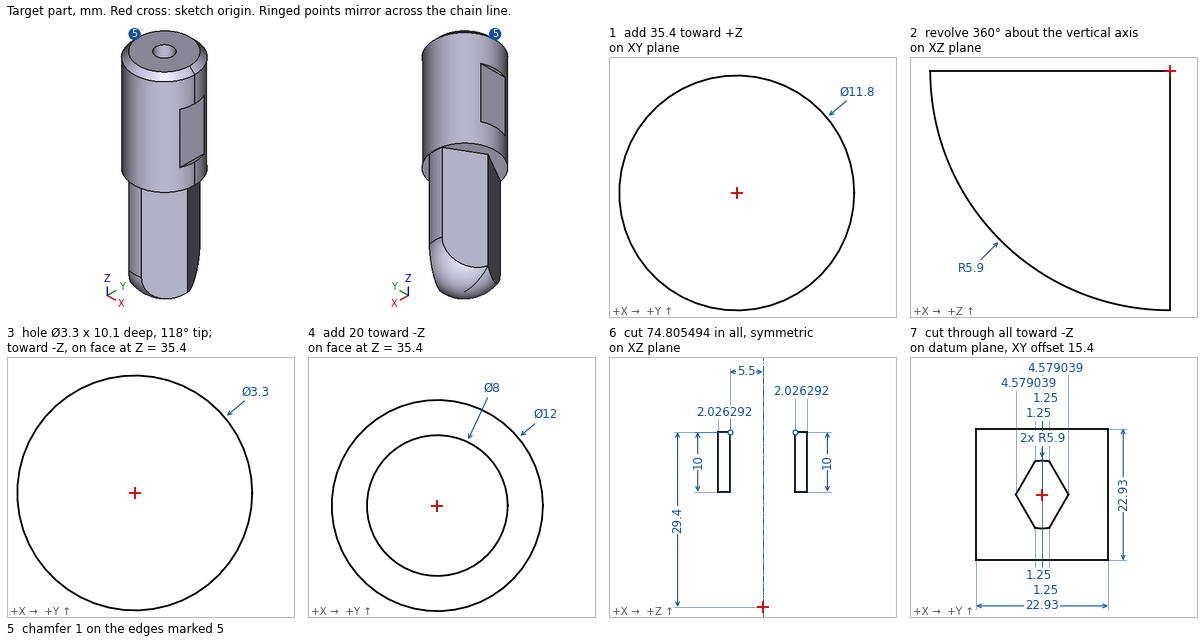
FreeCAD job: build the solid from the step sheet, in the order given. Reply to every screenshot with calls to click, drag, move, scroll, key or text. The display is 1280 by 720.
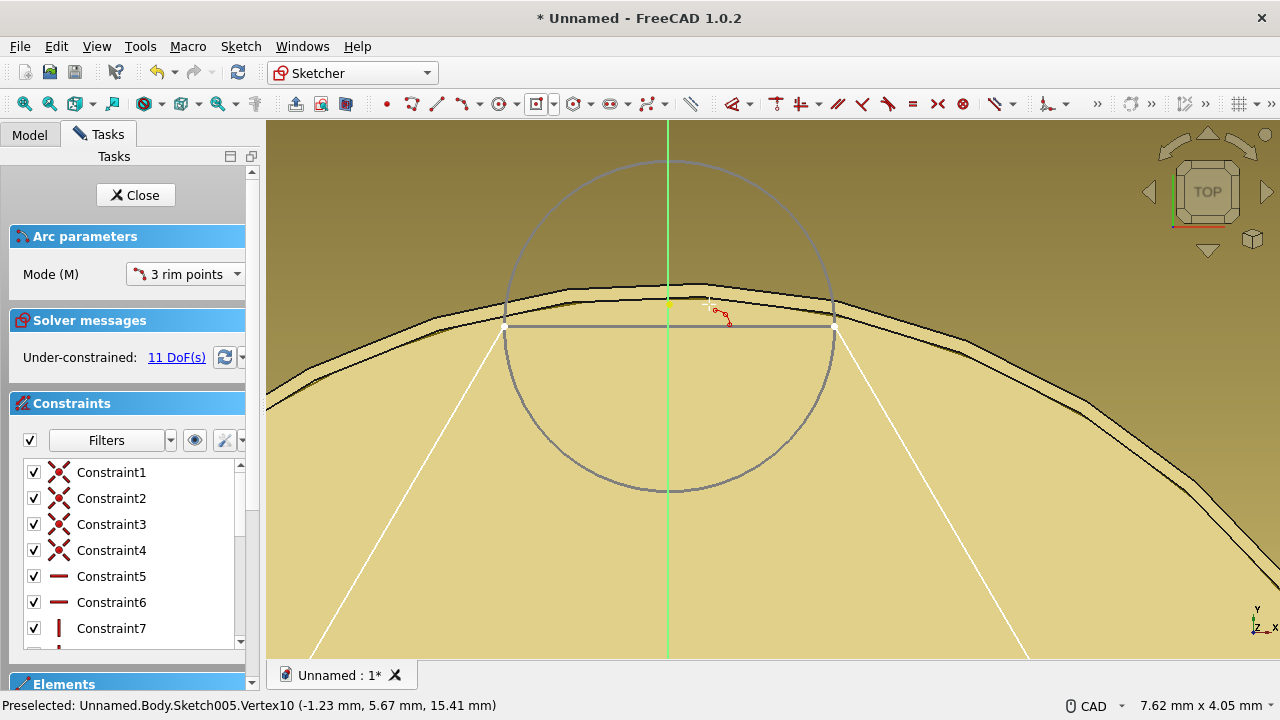
click(702, 297)
key(Escape)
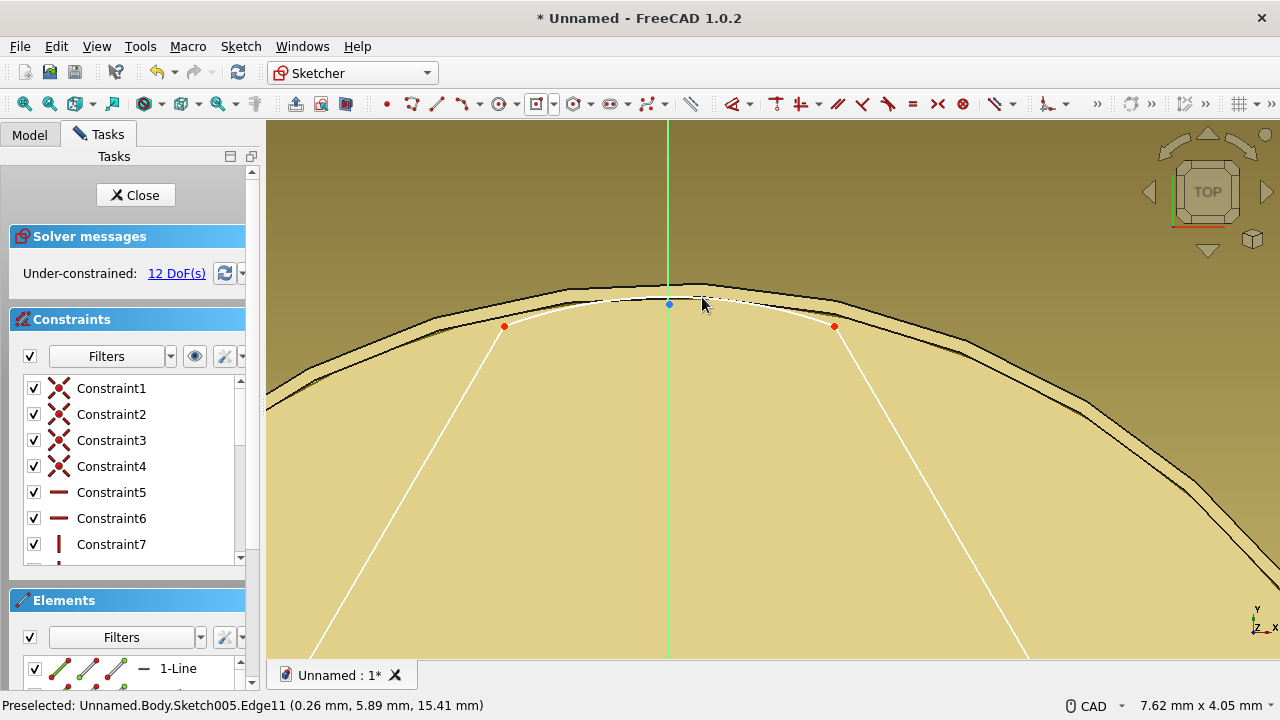
scroll(709, 303, down, 11)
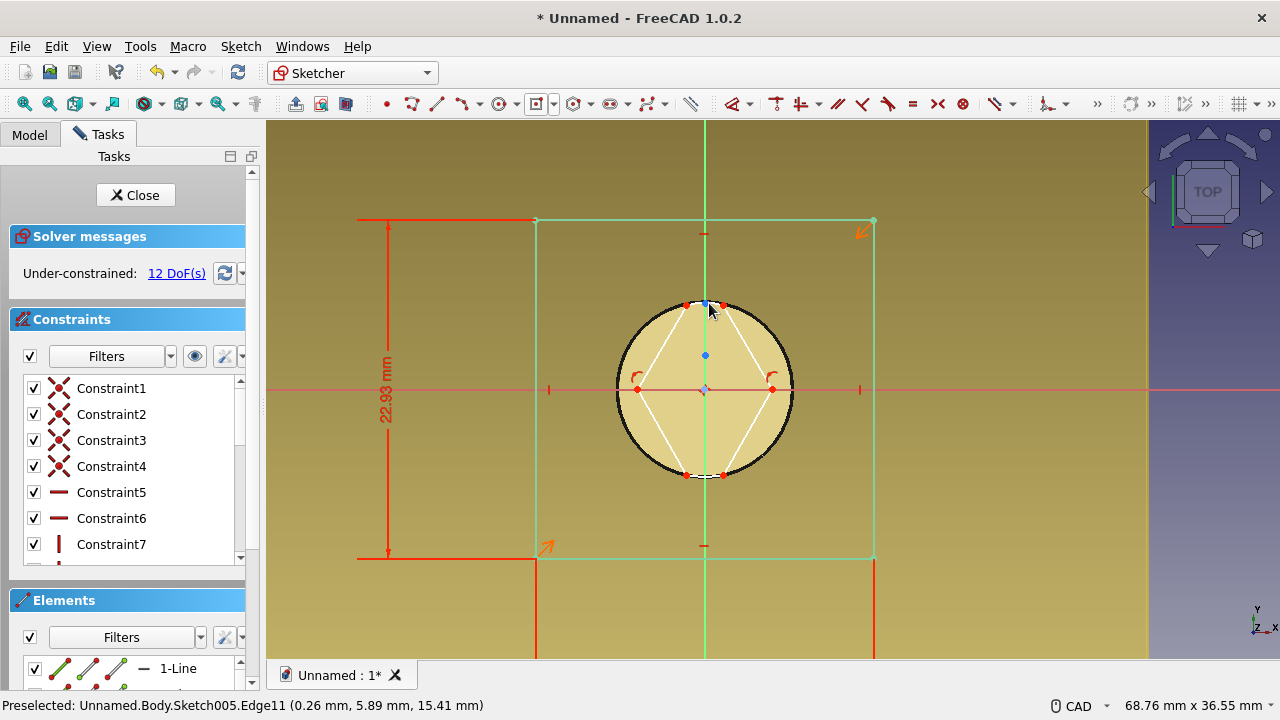
scroll(698, 476, up, 4)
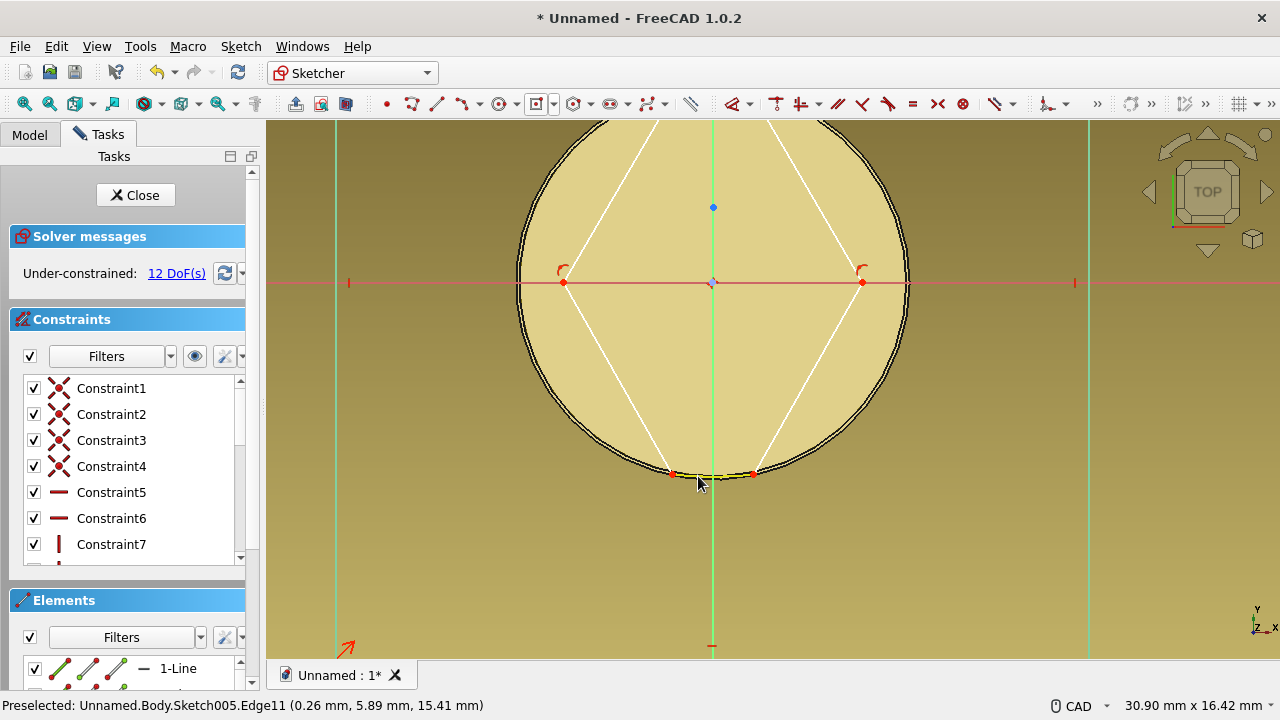
click(697, 476)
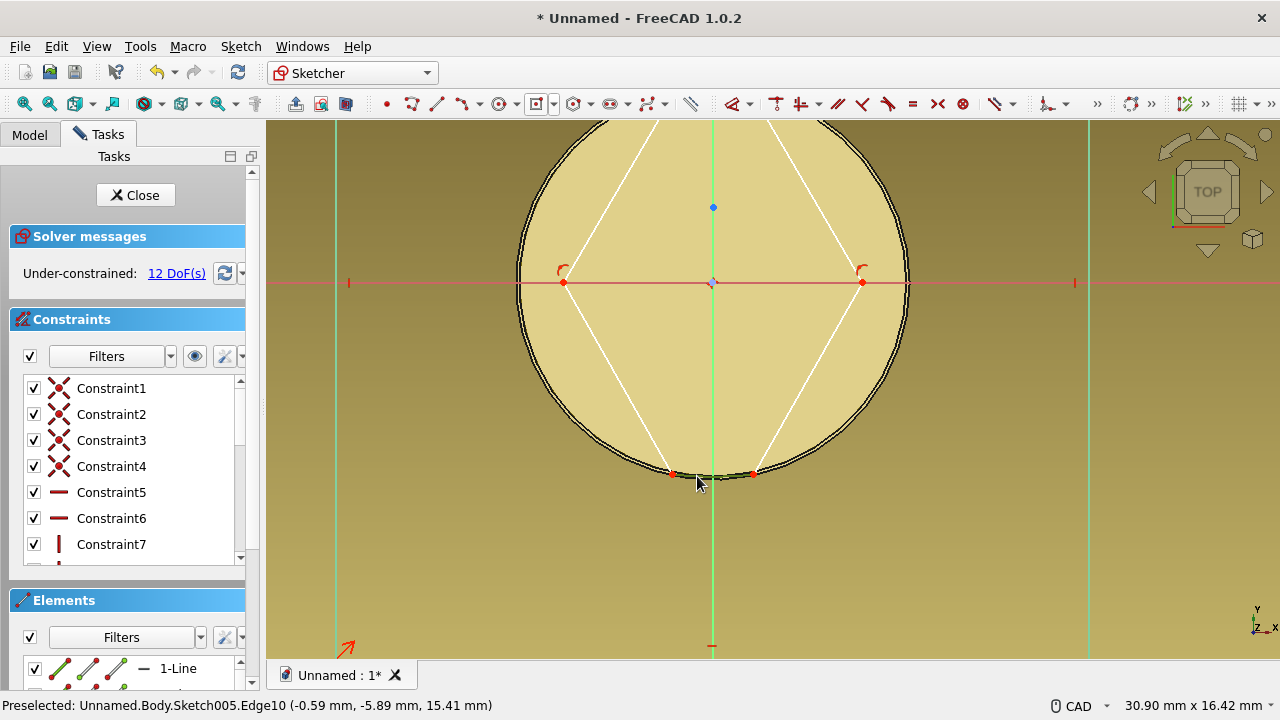
scroll(698, 477, down, 4)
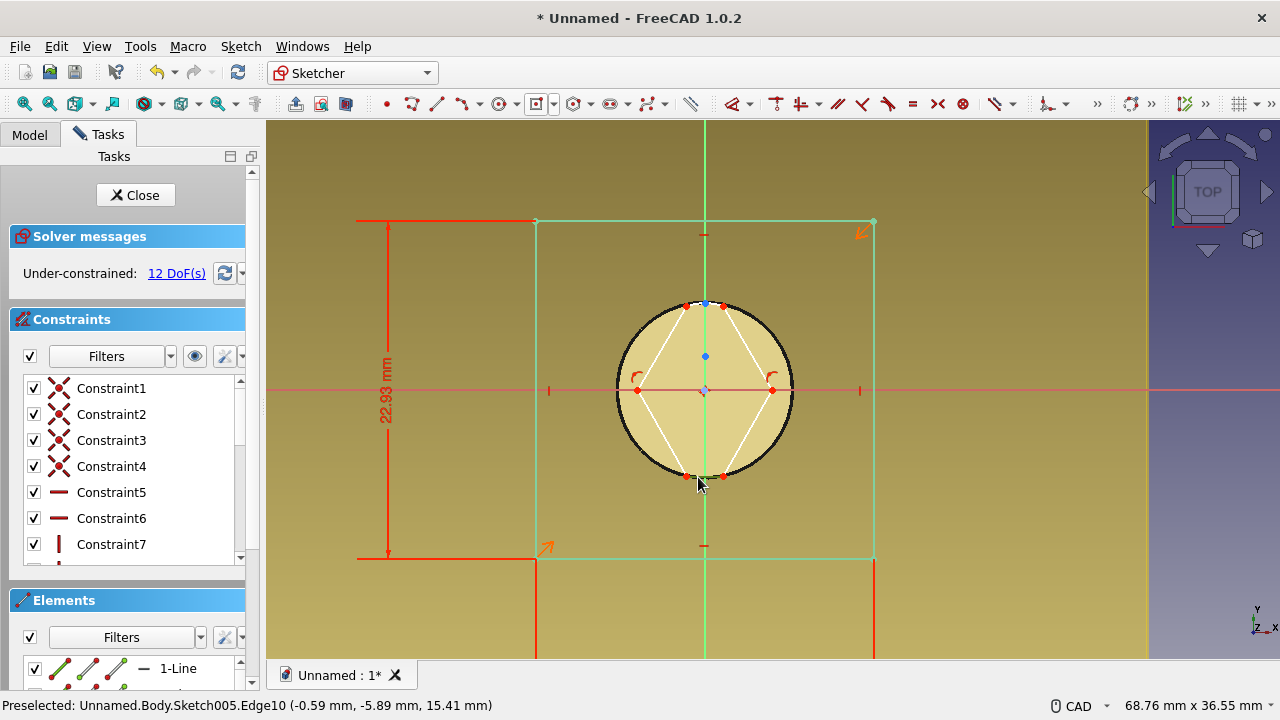
scroll(712, 304, up, 3)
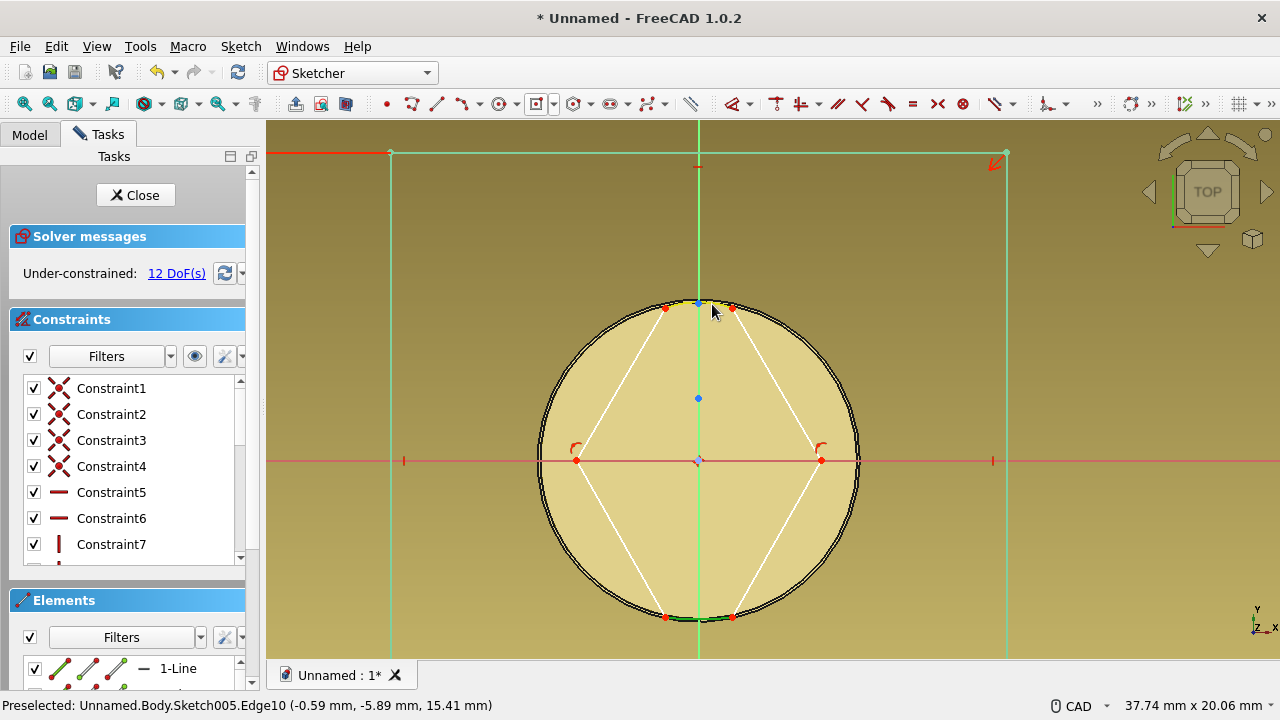
click(713, 303)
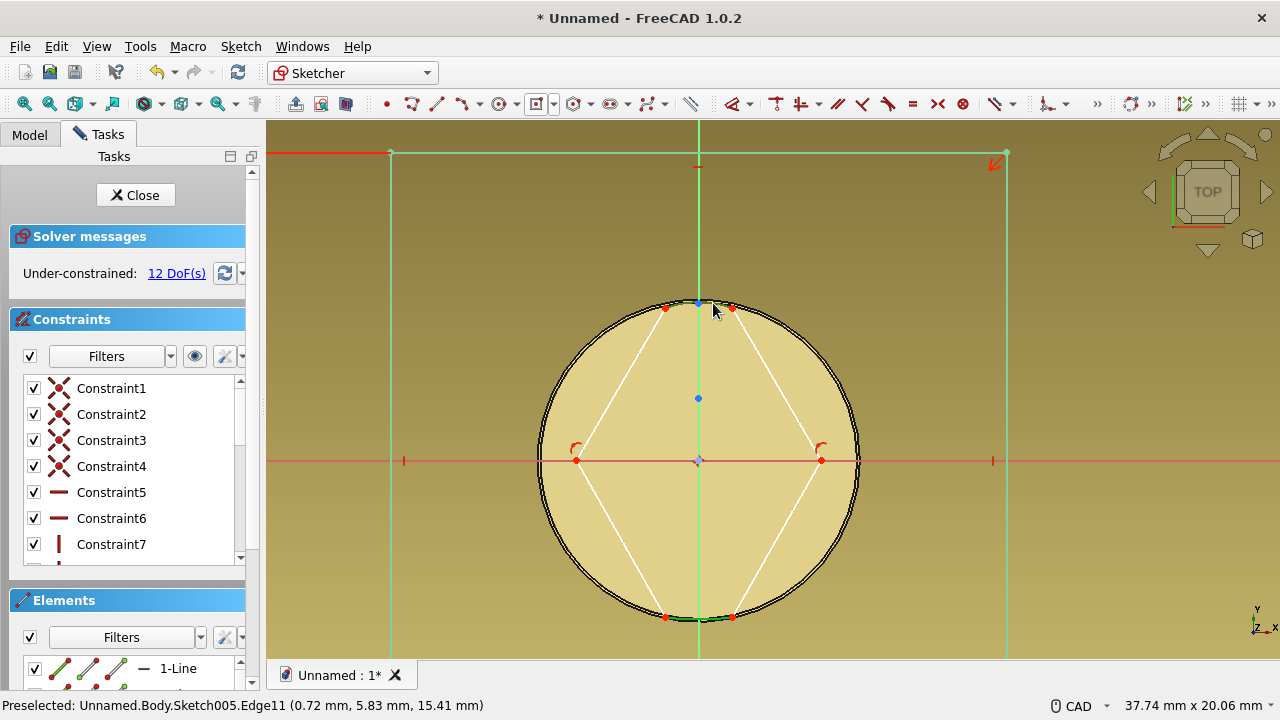
key(c)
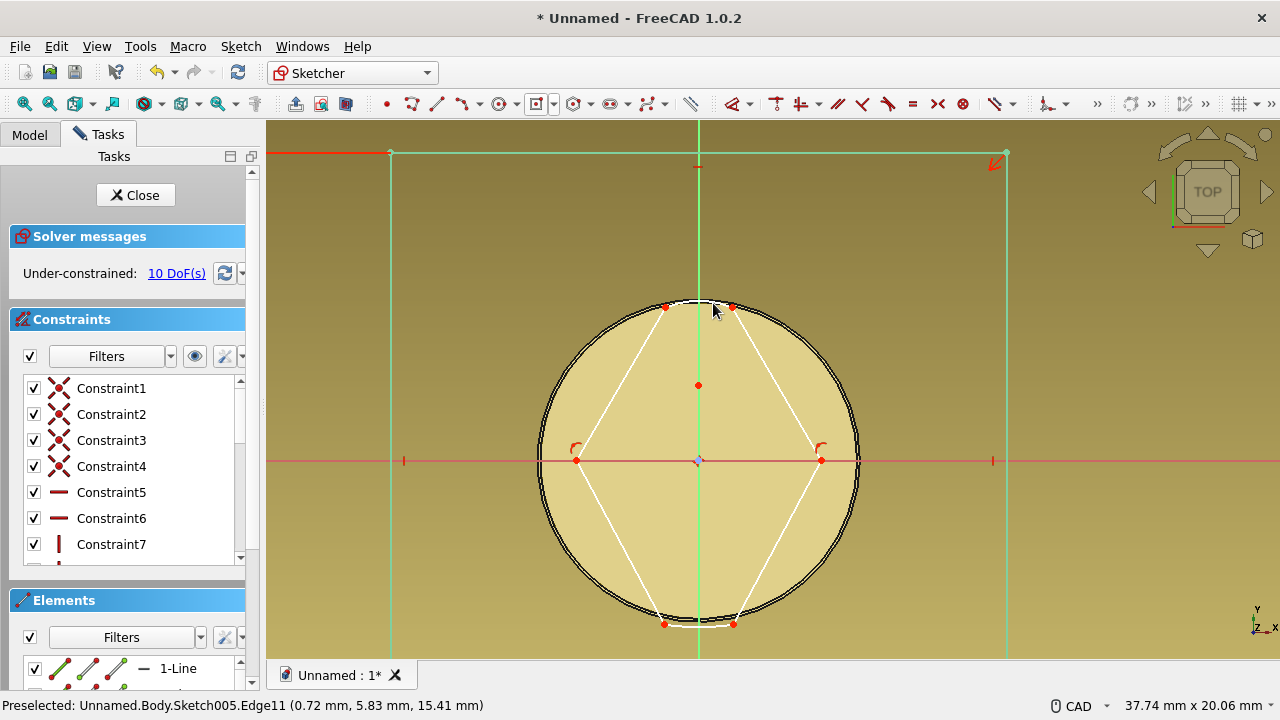
drag(689, 375, 709, 471)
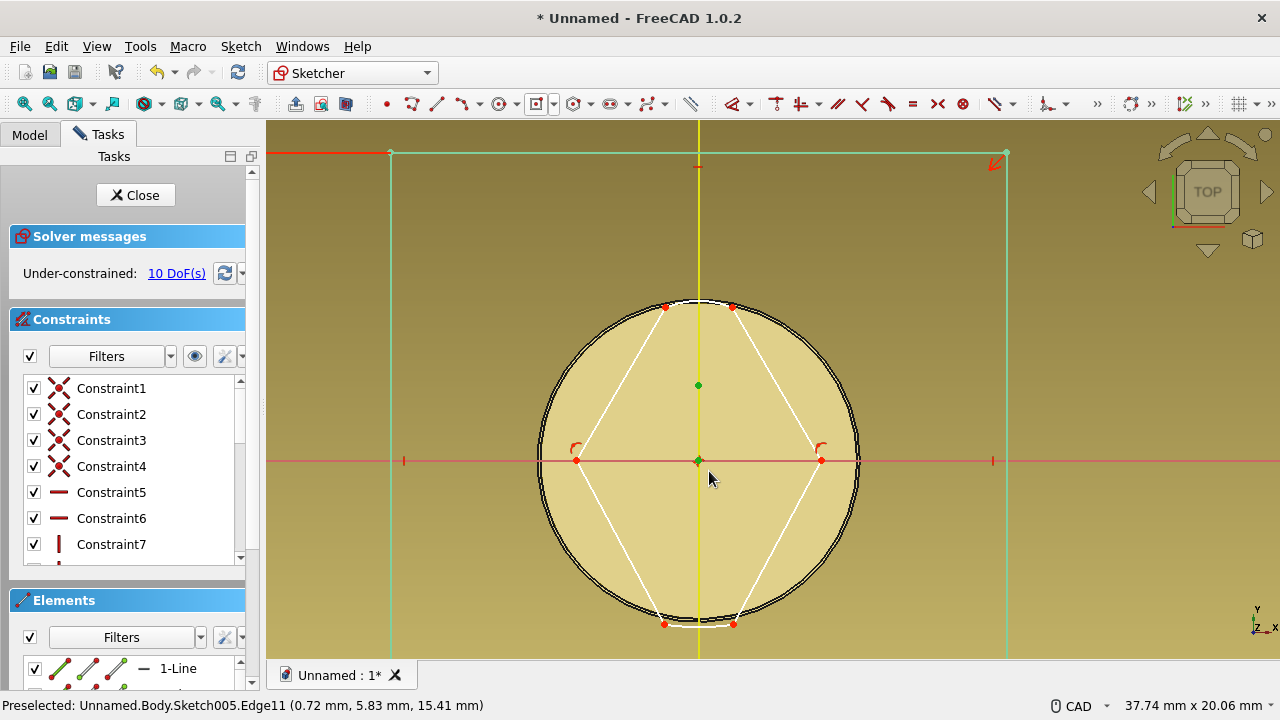
key(c)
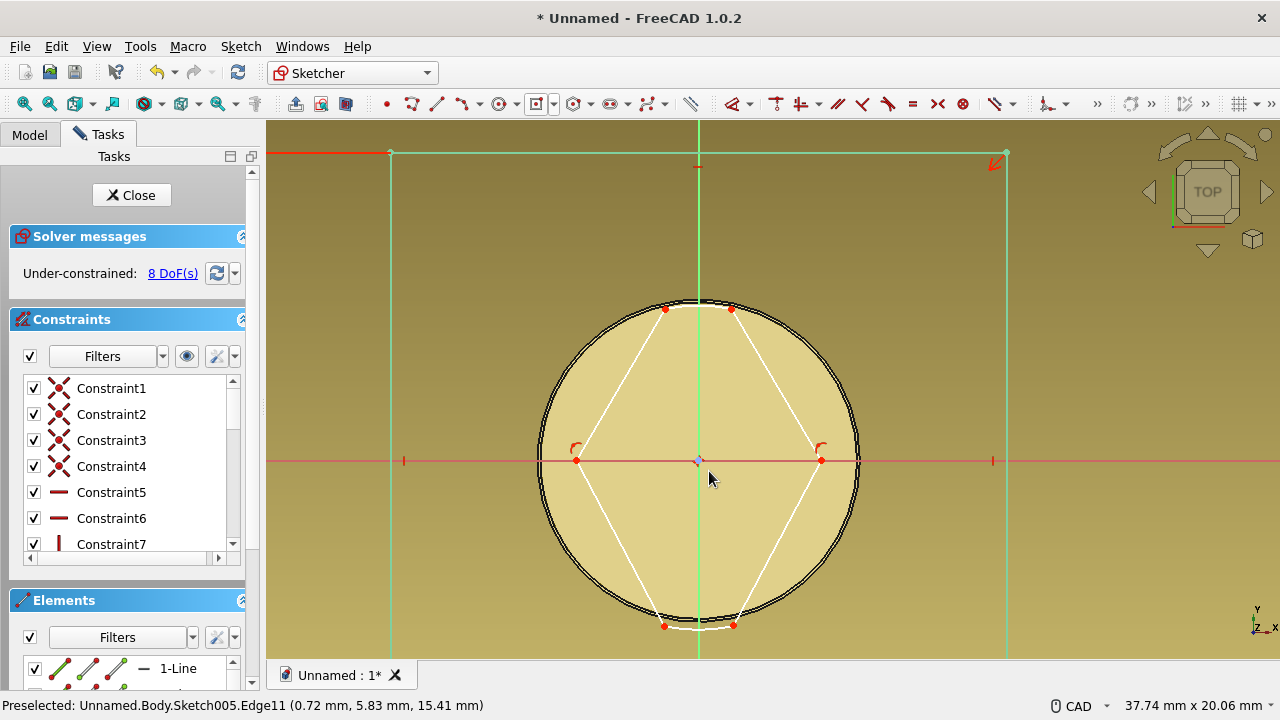
click(685, 629)